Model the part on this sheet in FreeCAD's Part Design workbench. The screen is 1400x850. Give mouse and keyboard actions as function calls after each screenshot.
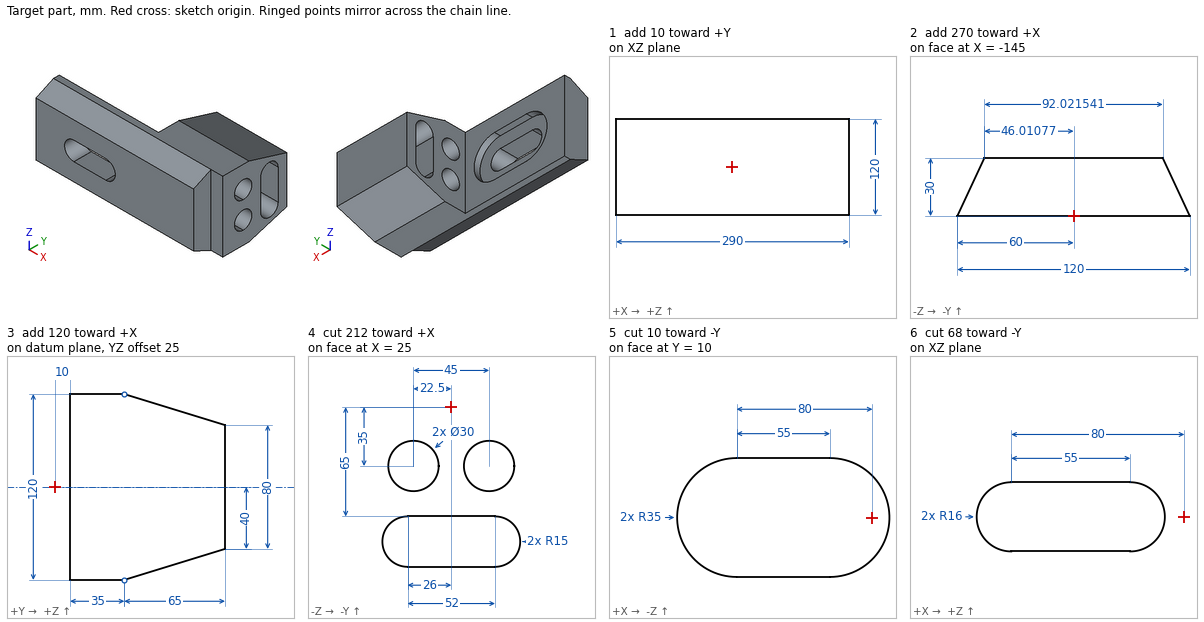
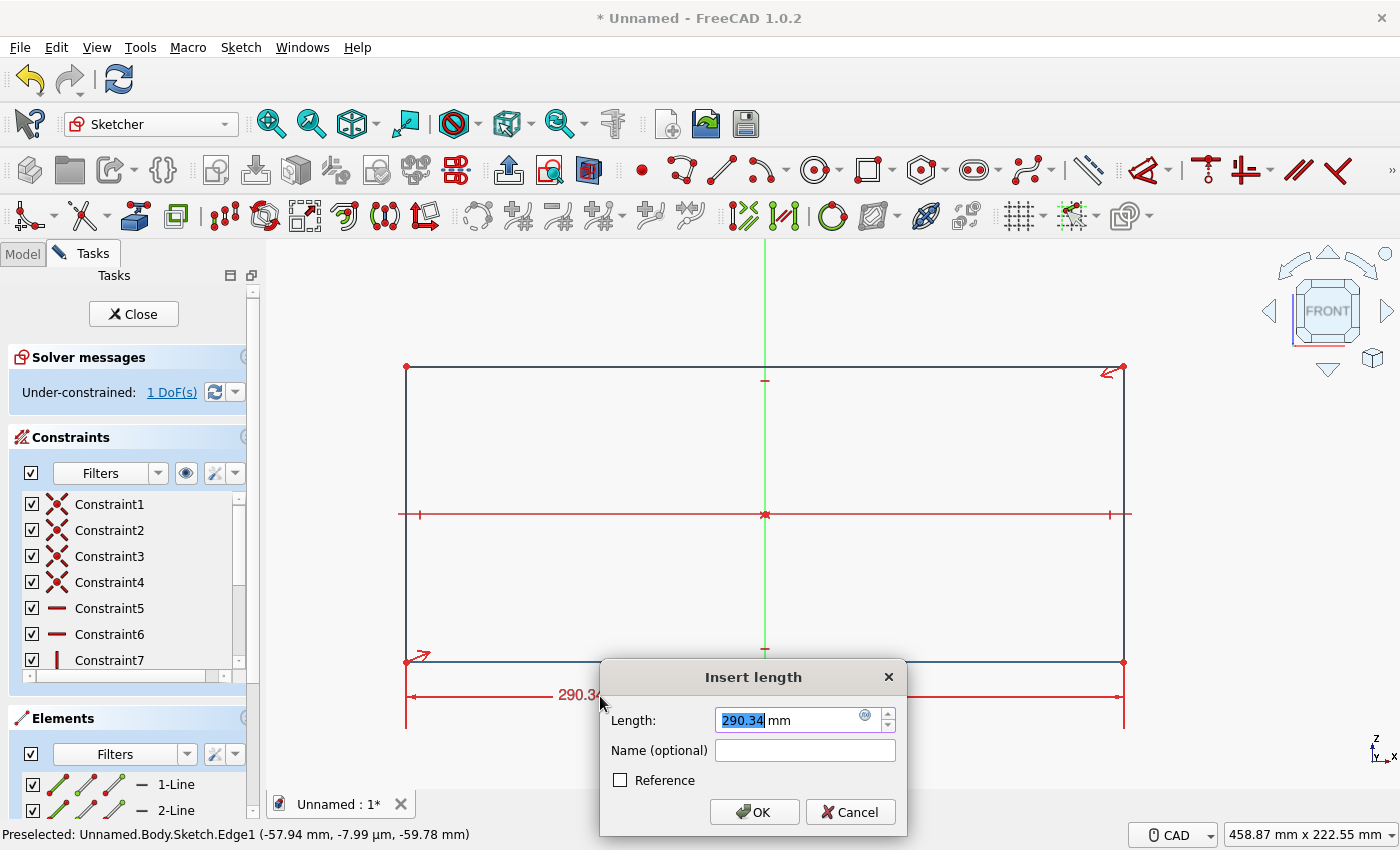
text(290)
key(Return)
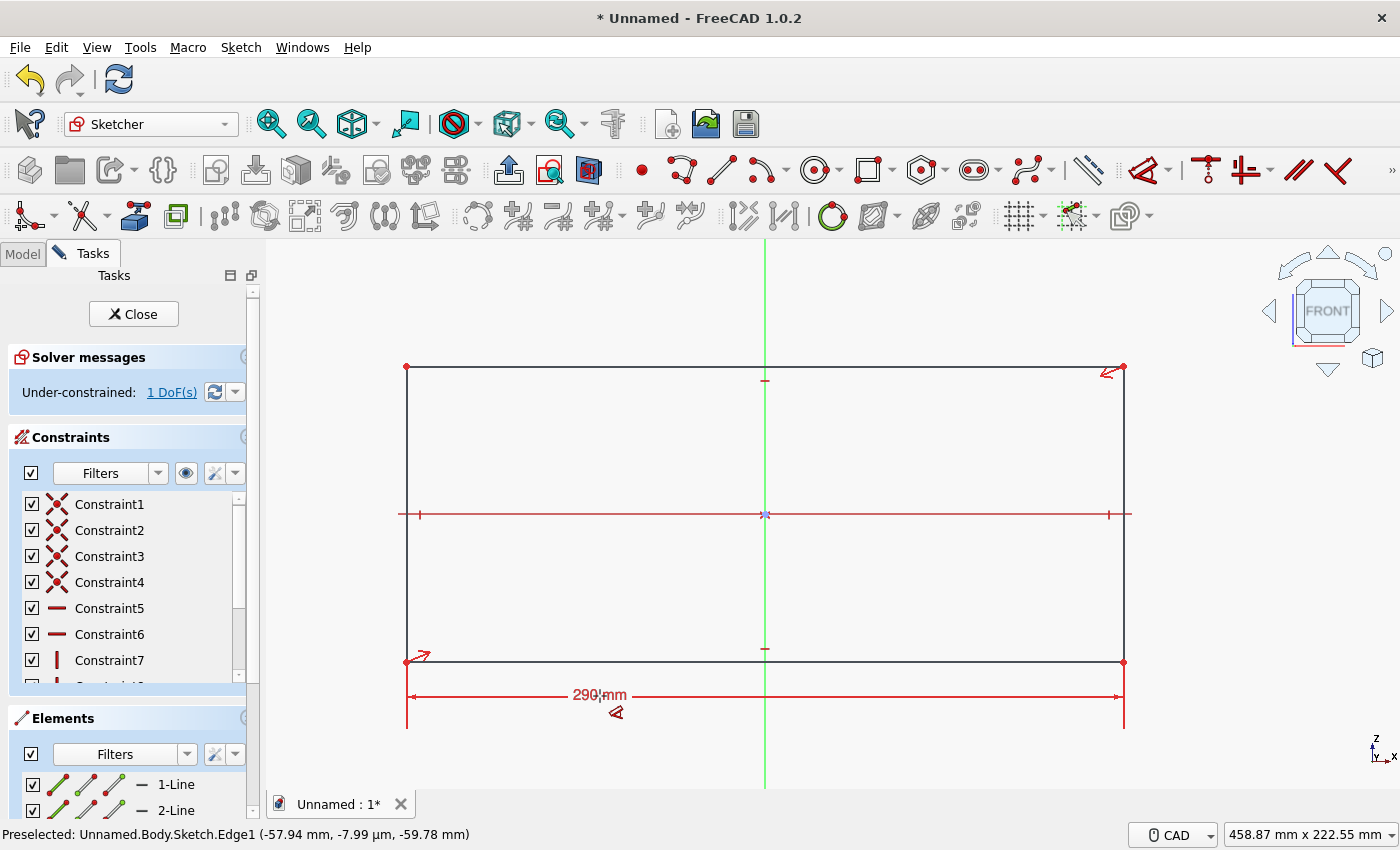
click(1124, 573)
click(1158, 446)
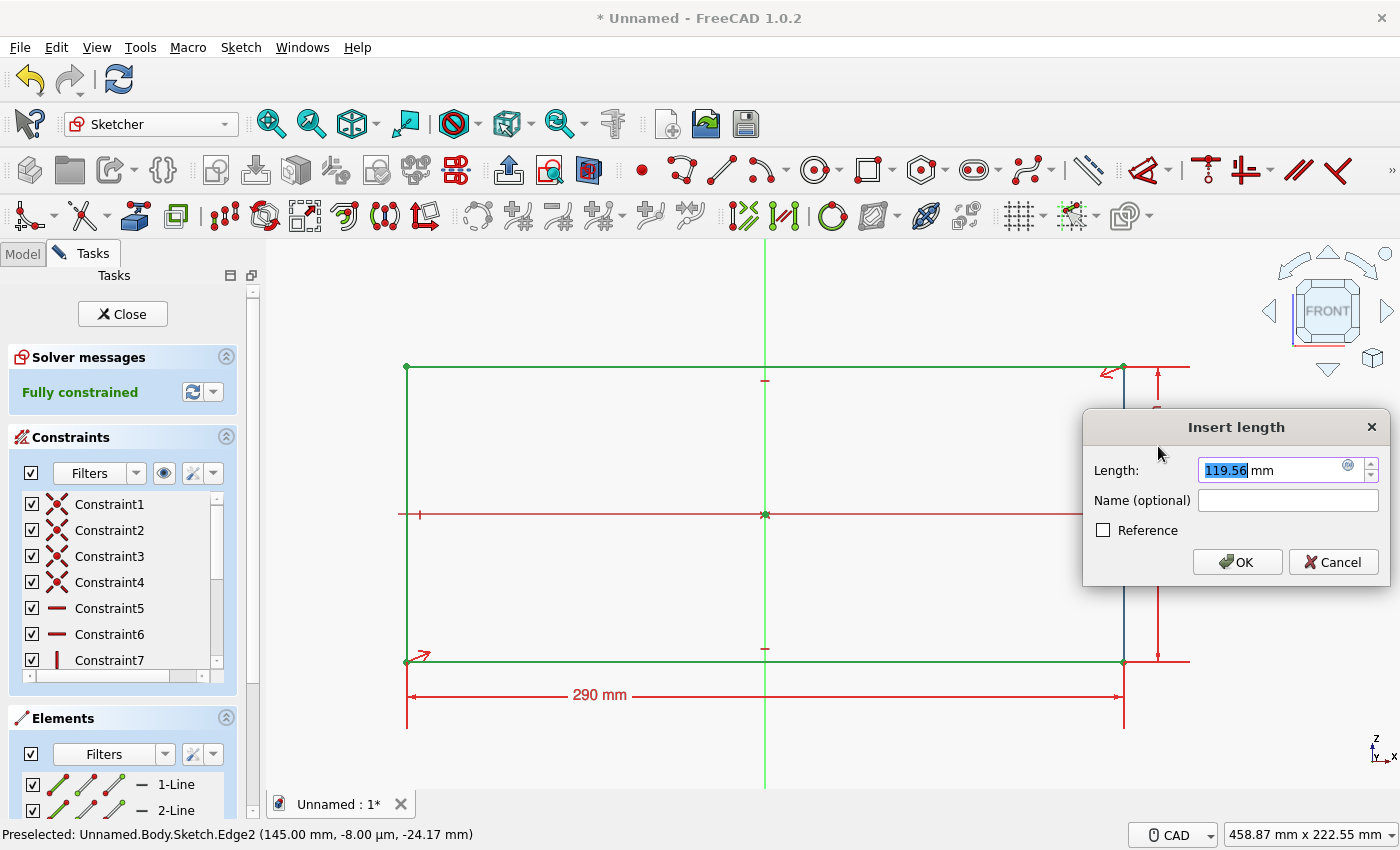
text(120)
key(Return)
key(Escape)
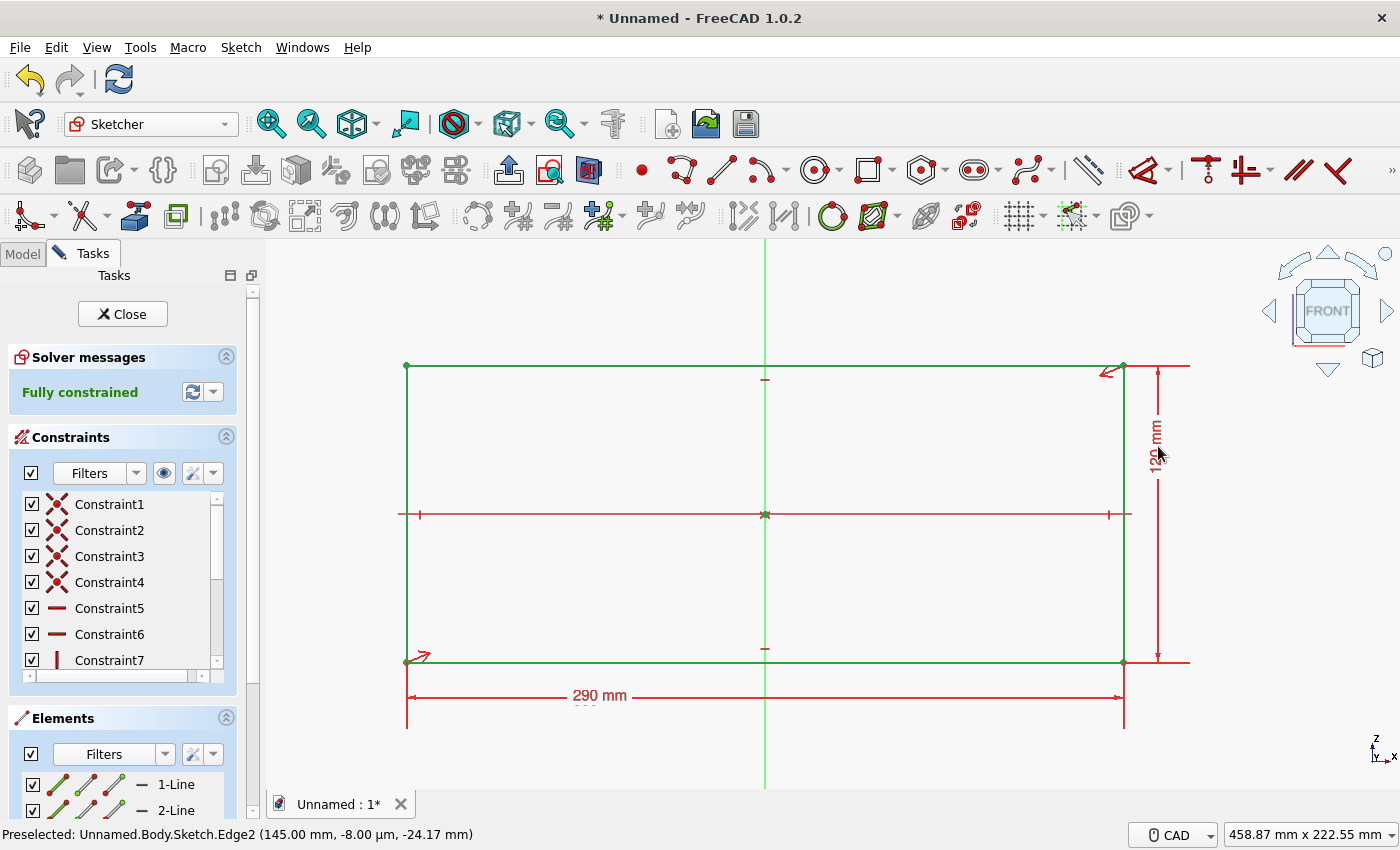
click(123, 314)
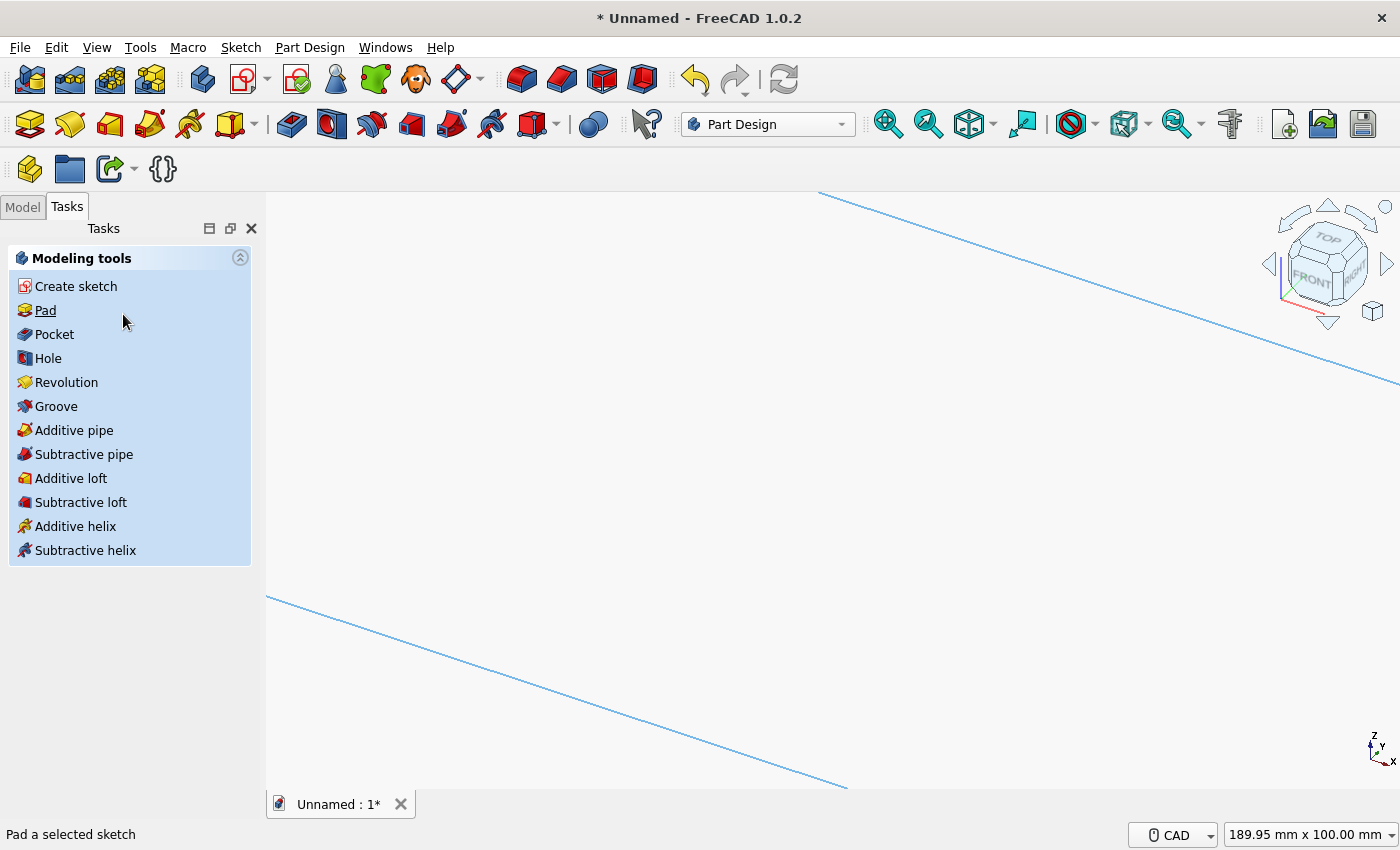
click(30, 124)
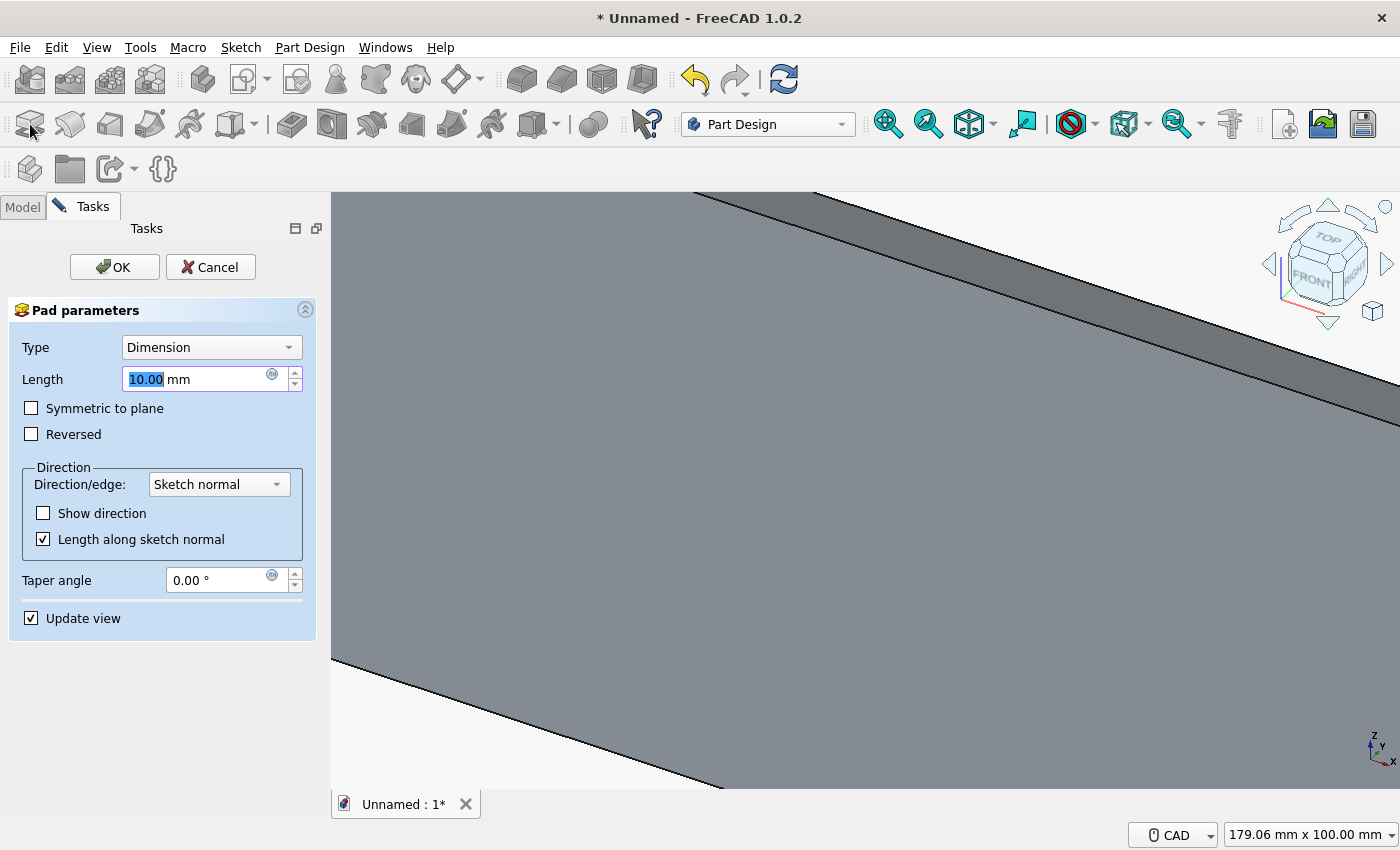
text(10)
key(Tab)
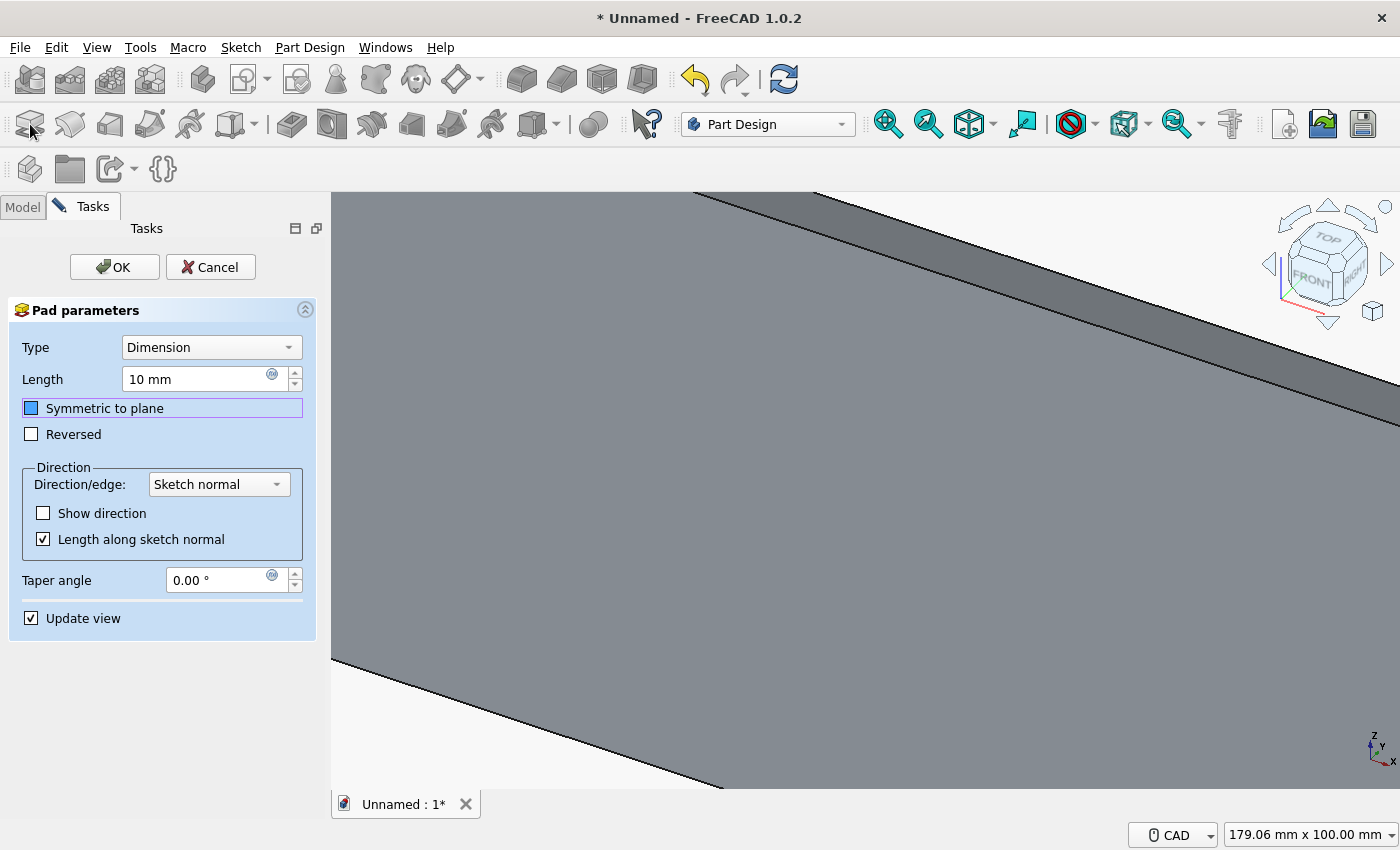
click(30, 434)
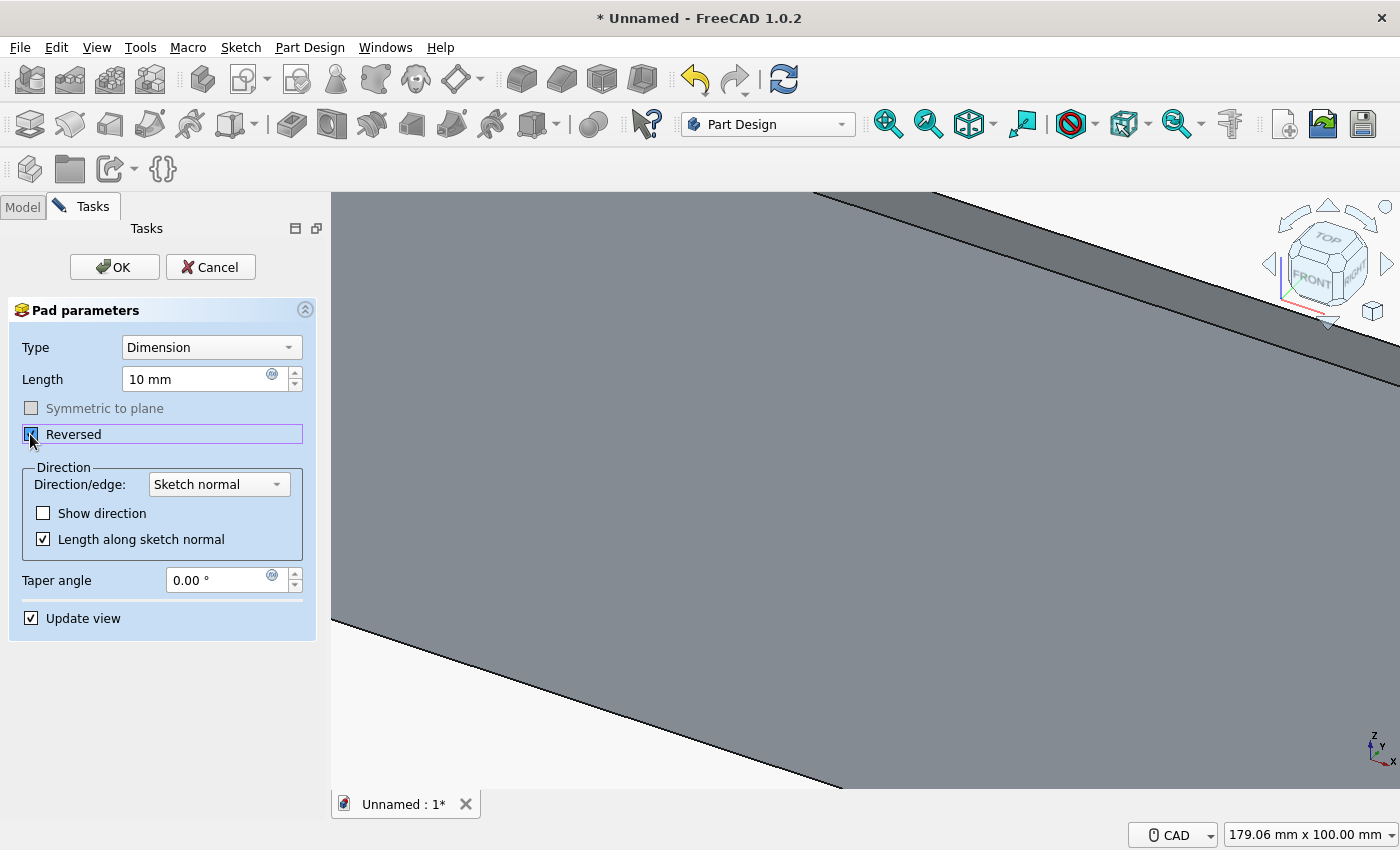
click(115, 267)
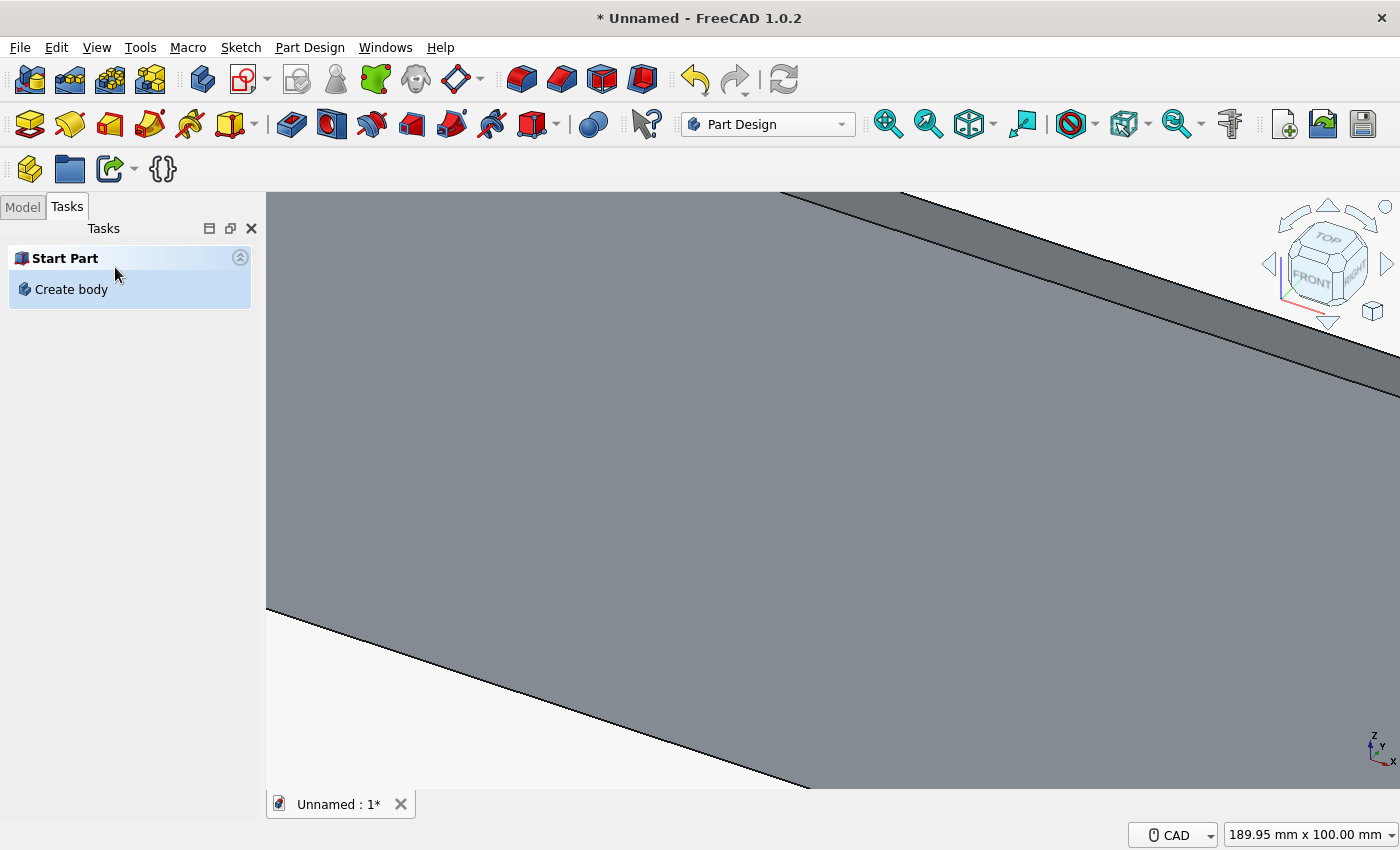
key(v)
key(f)